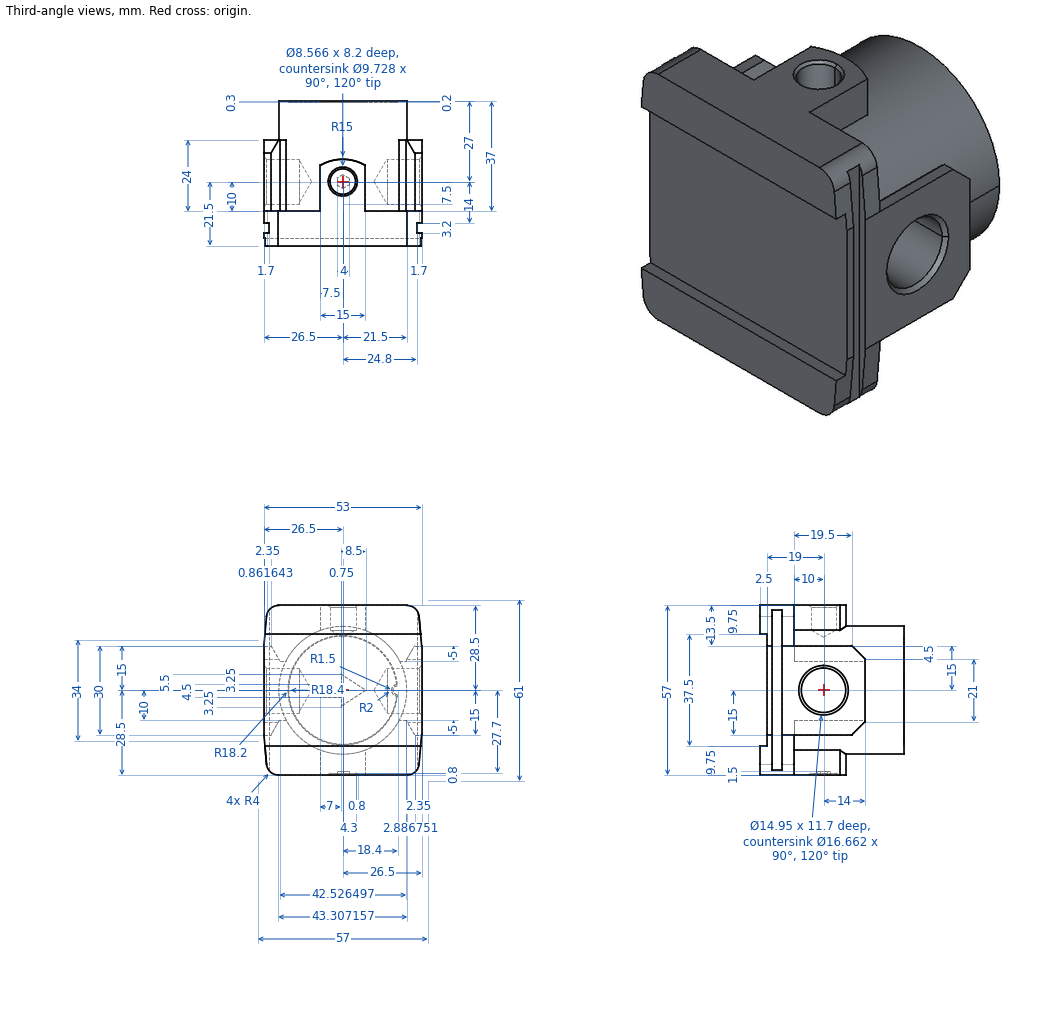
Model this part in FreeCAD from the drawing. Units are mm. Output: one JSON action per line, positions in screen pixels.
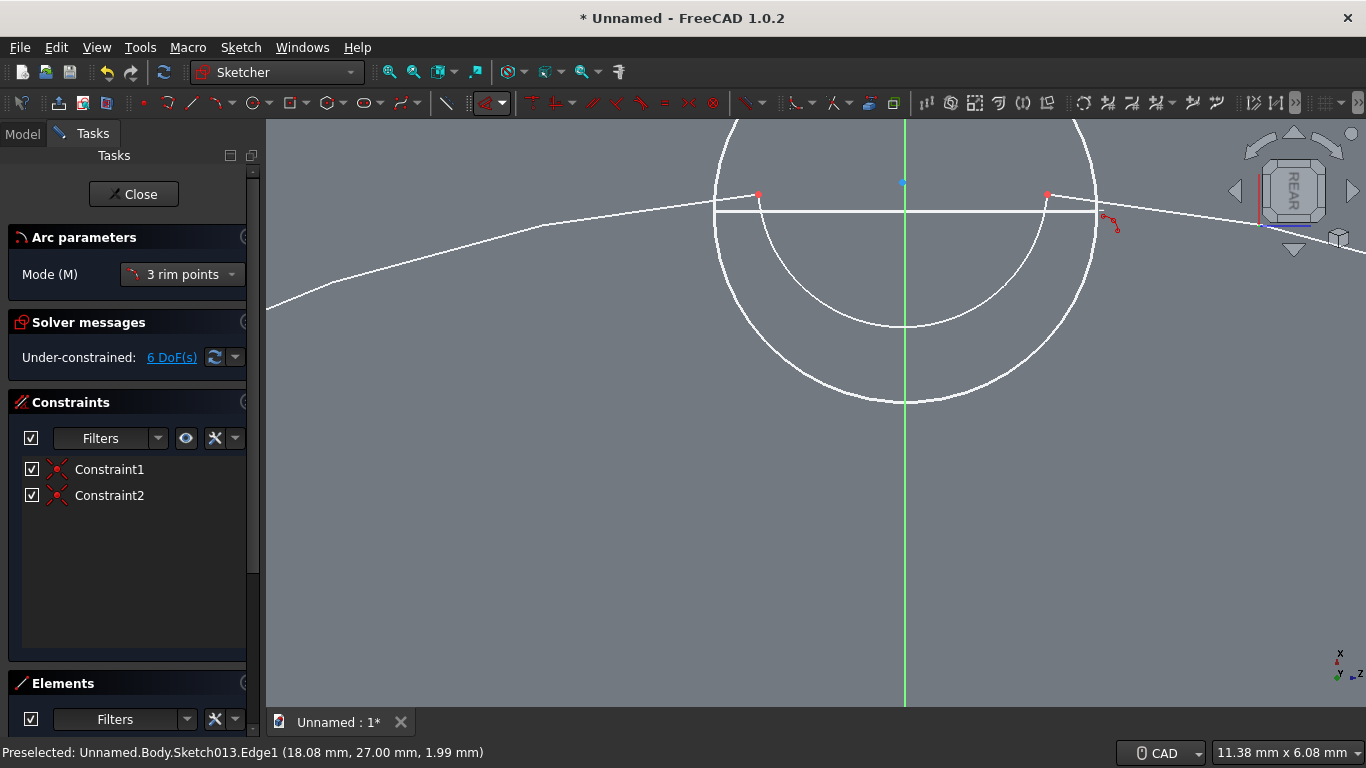
{"action": "scroll", "coordinate": [728, 220], "scroll_direction": "down", "scroll_amount": 11}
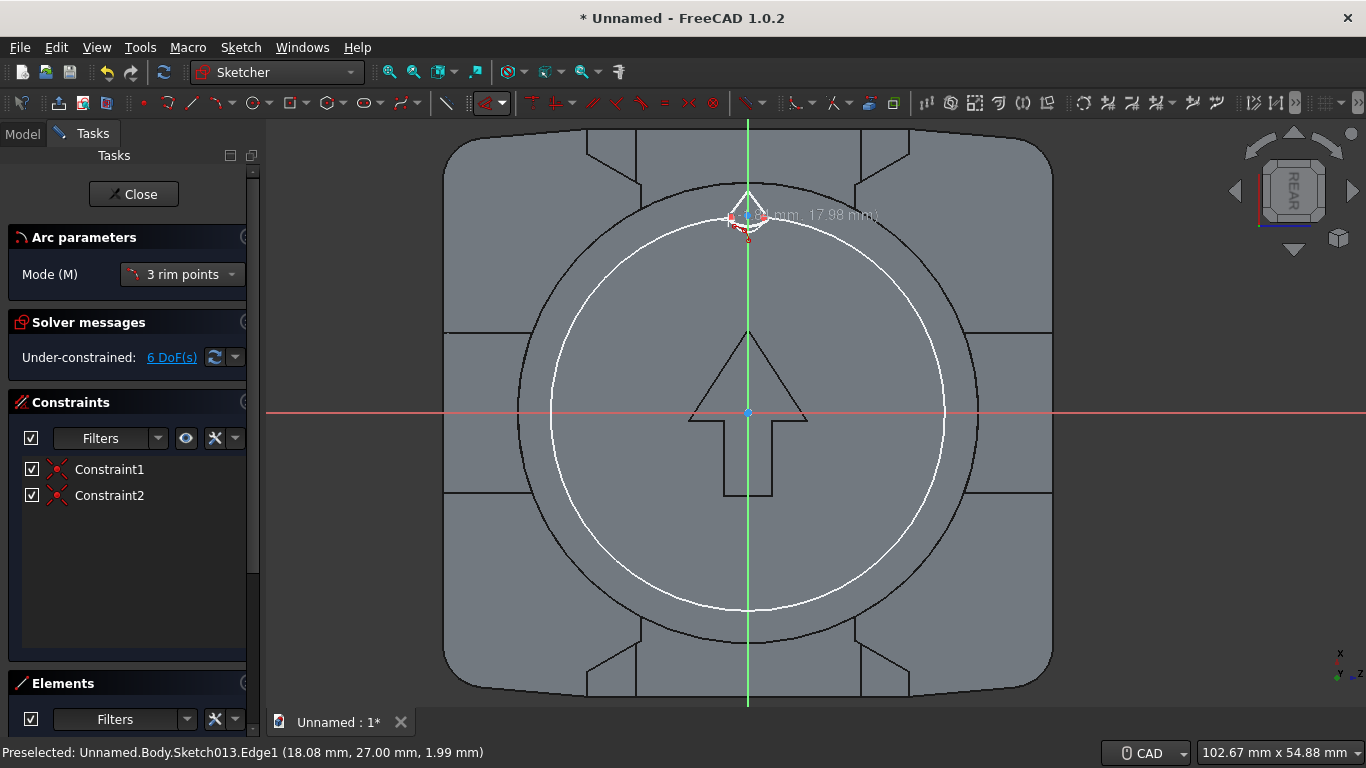
{"action": "scroll", "coordinate": [637, 573], "scroll_direction": "up", "scroll_amount": 11}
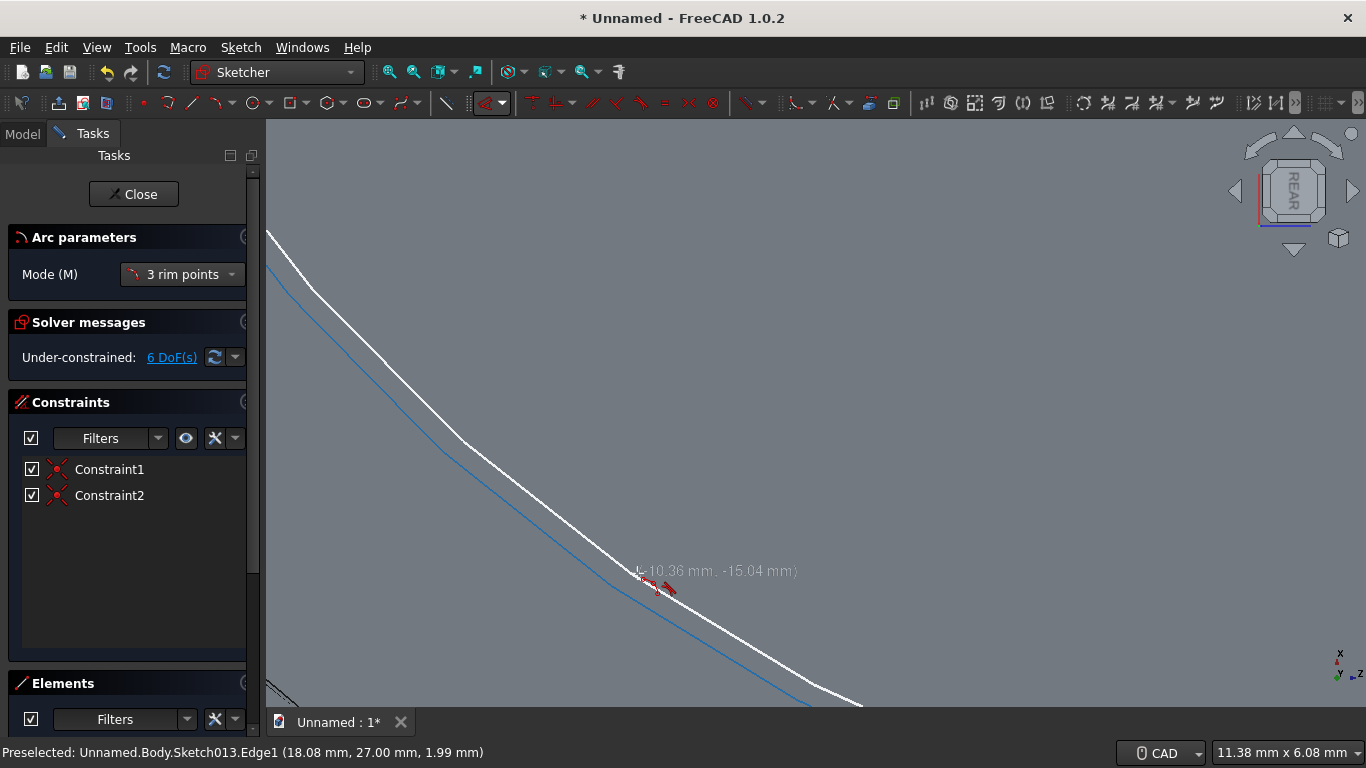
{"action": "left_click", "coordinate": [633, 568]}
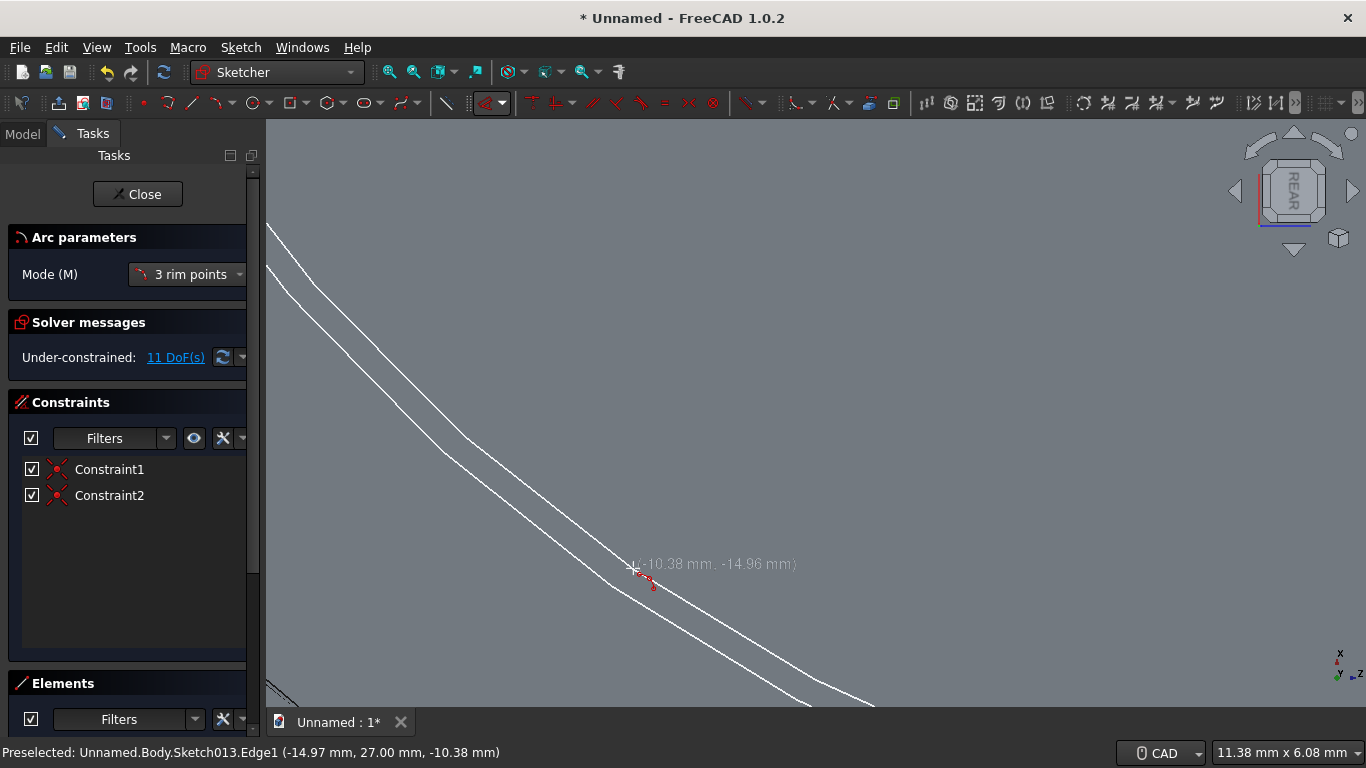
{"action": "scroll", "coordinate": [637, 574], "scroll_direction": "down", "scroll_amount": 11}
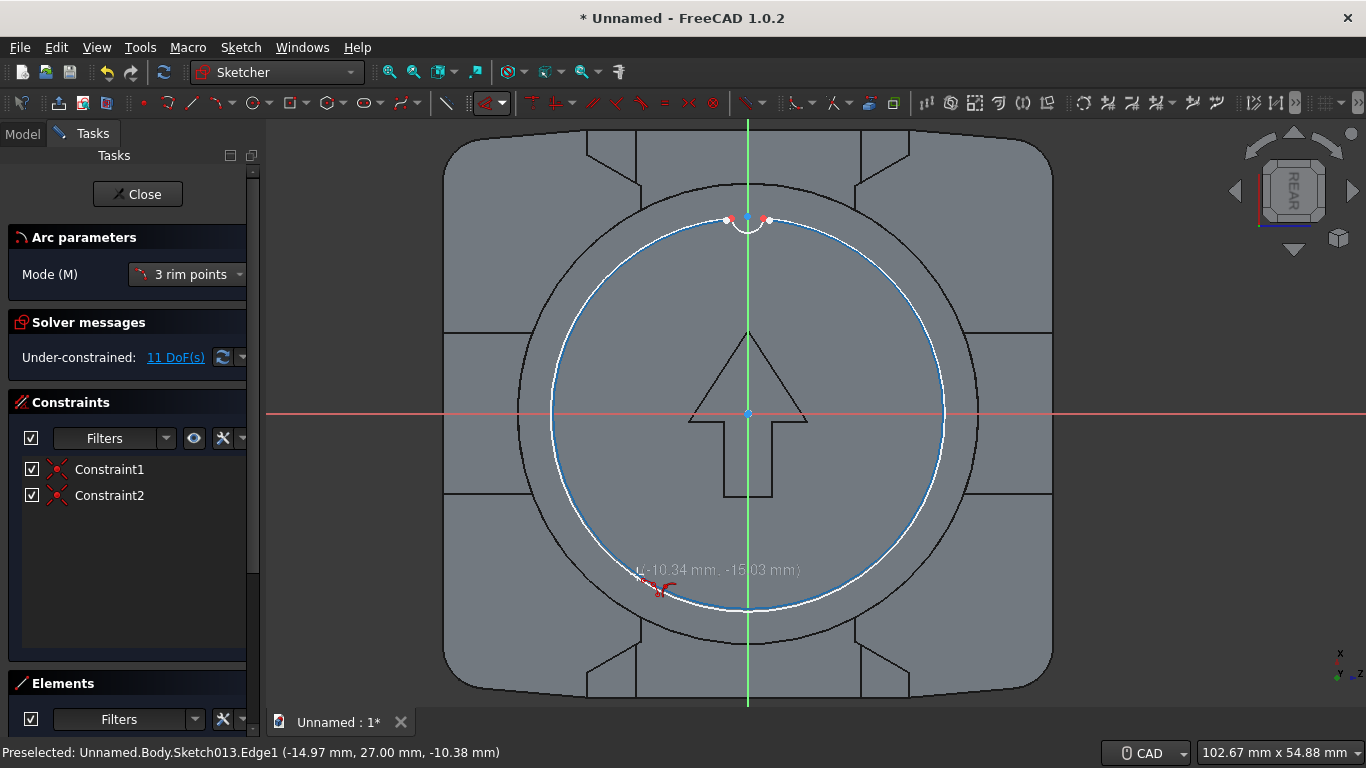
{"action": "scroll", "coordinate": [769, 220], "scroll_direction": "up", "scroll_amount": 11}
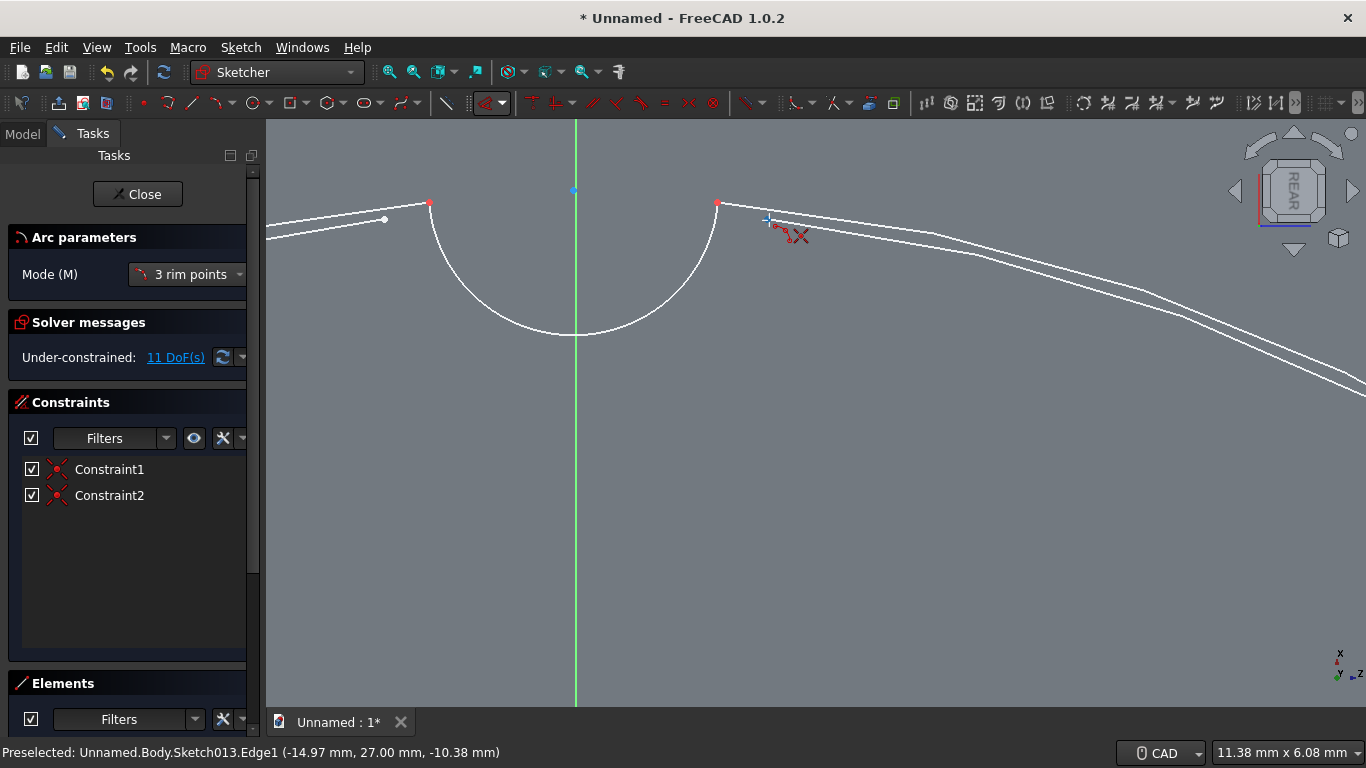
{"action": "left_click", "coordinate": [768, 219]}
{"action": "left_click", "coordinate": [385, 219]}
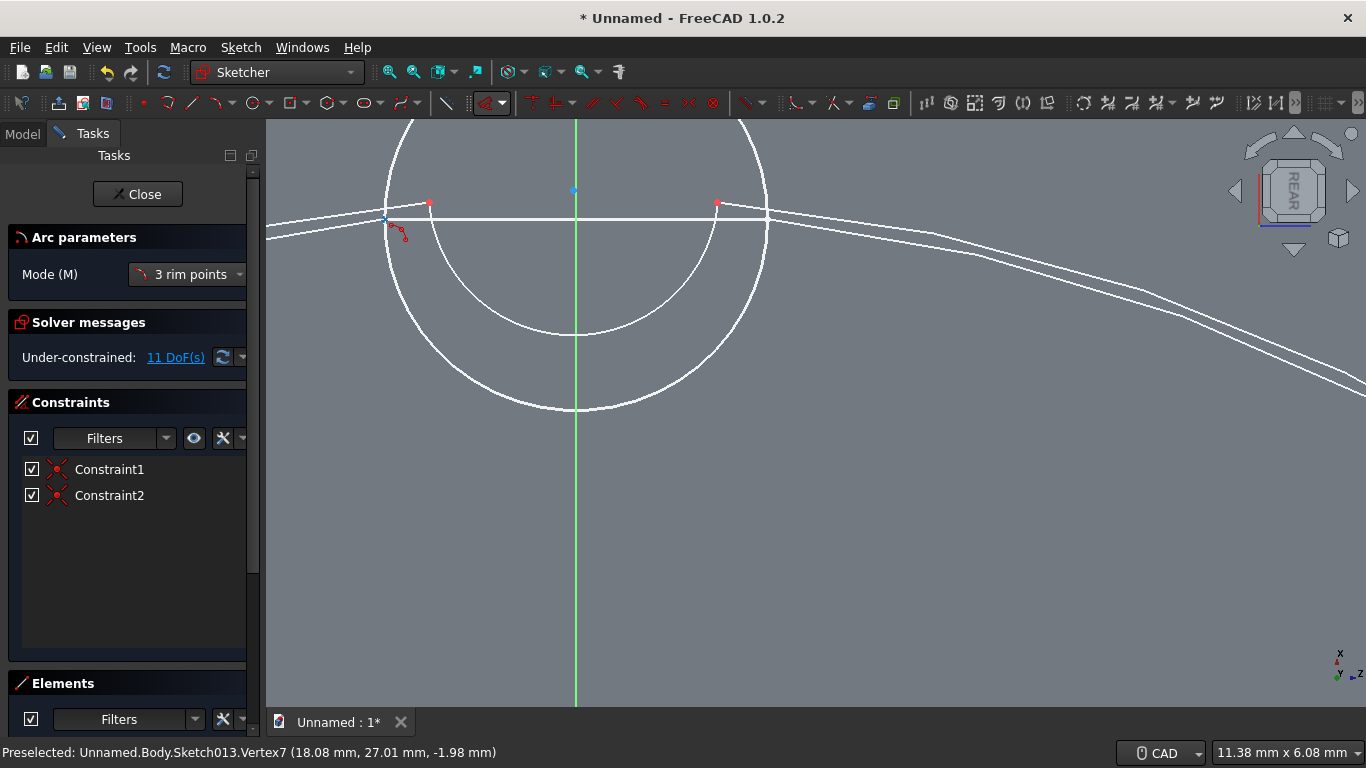
{"action": "scroll", "coordinate": [769, 219], "scroll_direction": "down", "scroll_amount": 11}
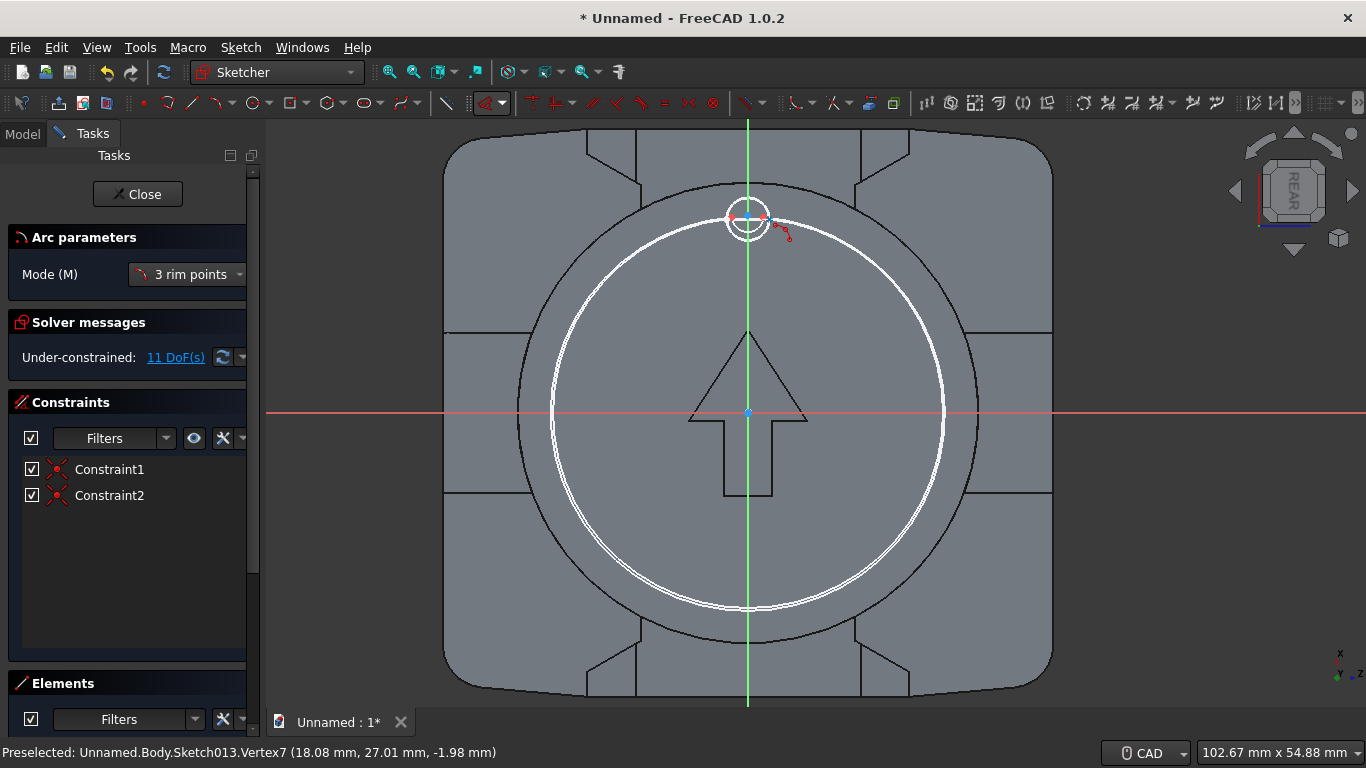
{"action": "scroll", "coordinate": [737, 234], "scroll_direction": "up", "scroll_amount": 6}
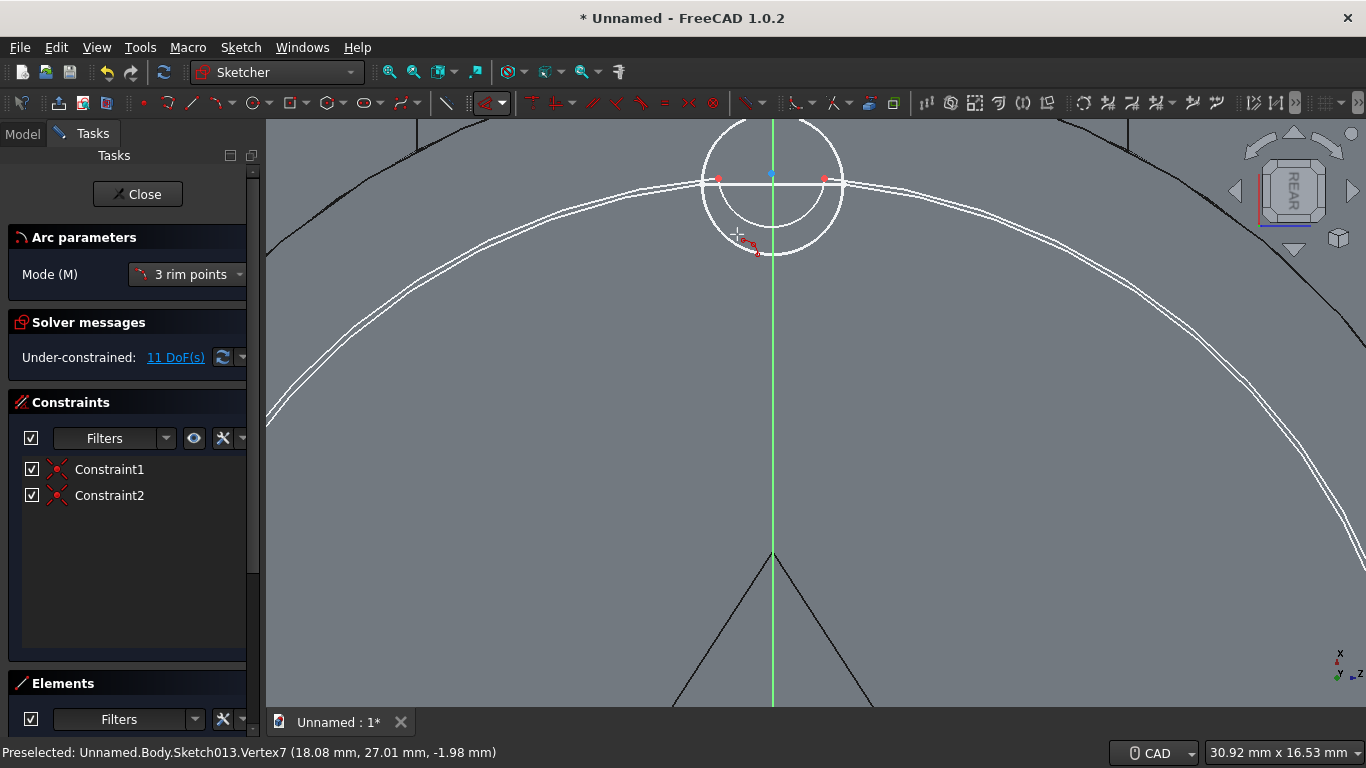
{"action": "left_click", "coordinate": [734, 233]}
{"action": "key", "text": "Escape"}